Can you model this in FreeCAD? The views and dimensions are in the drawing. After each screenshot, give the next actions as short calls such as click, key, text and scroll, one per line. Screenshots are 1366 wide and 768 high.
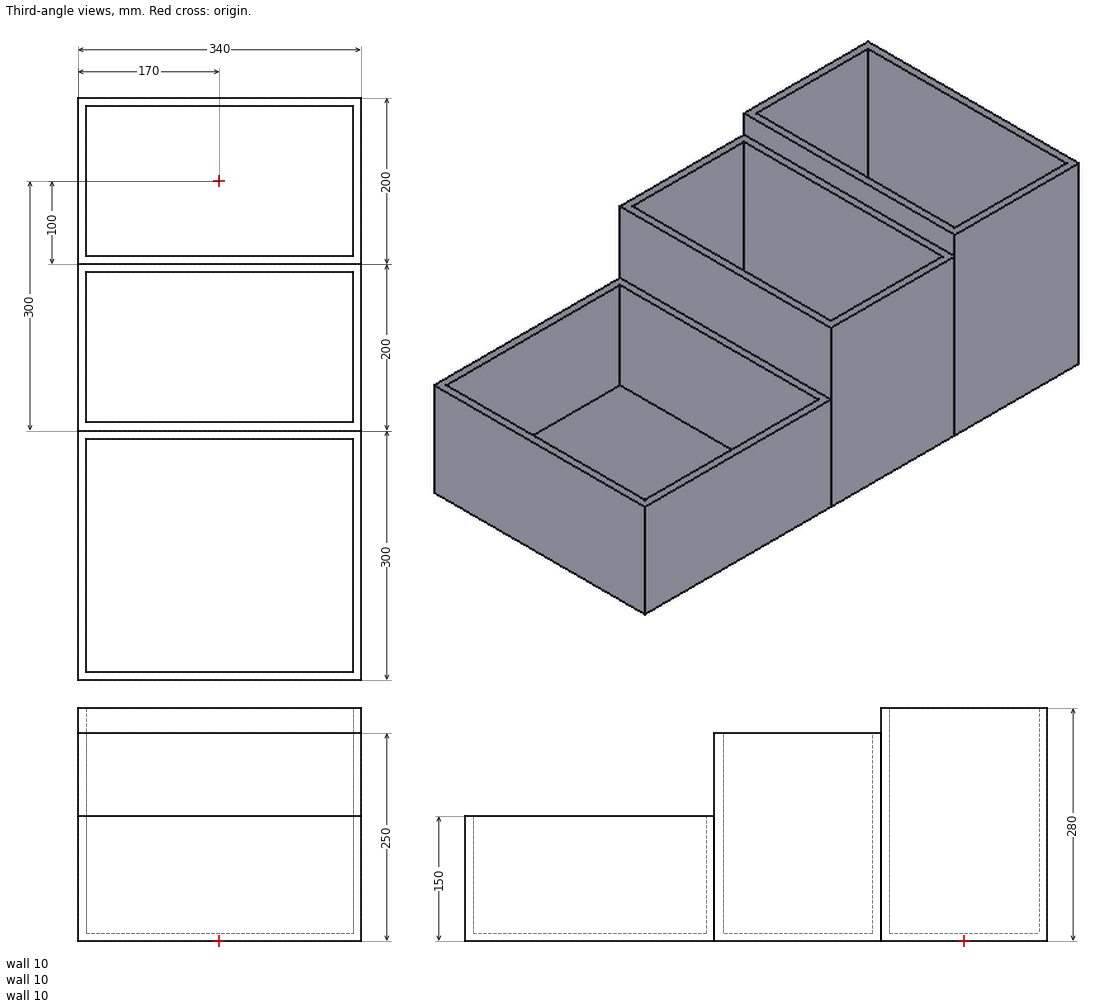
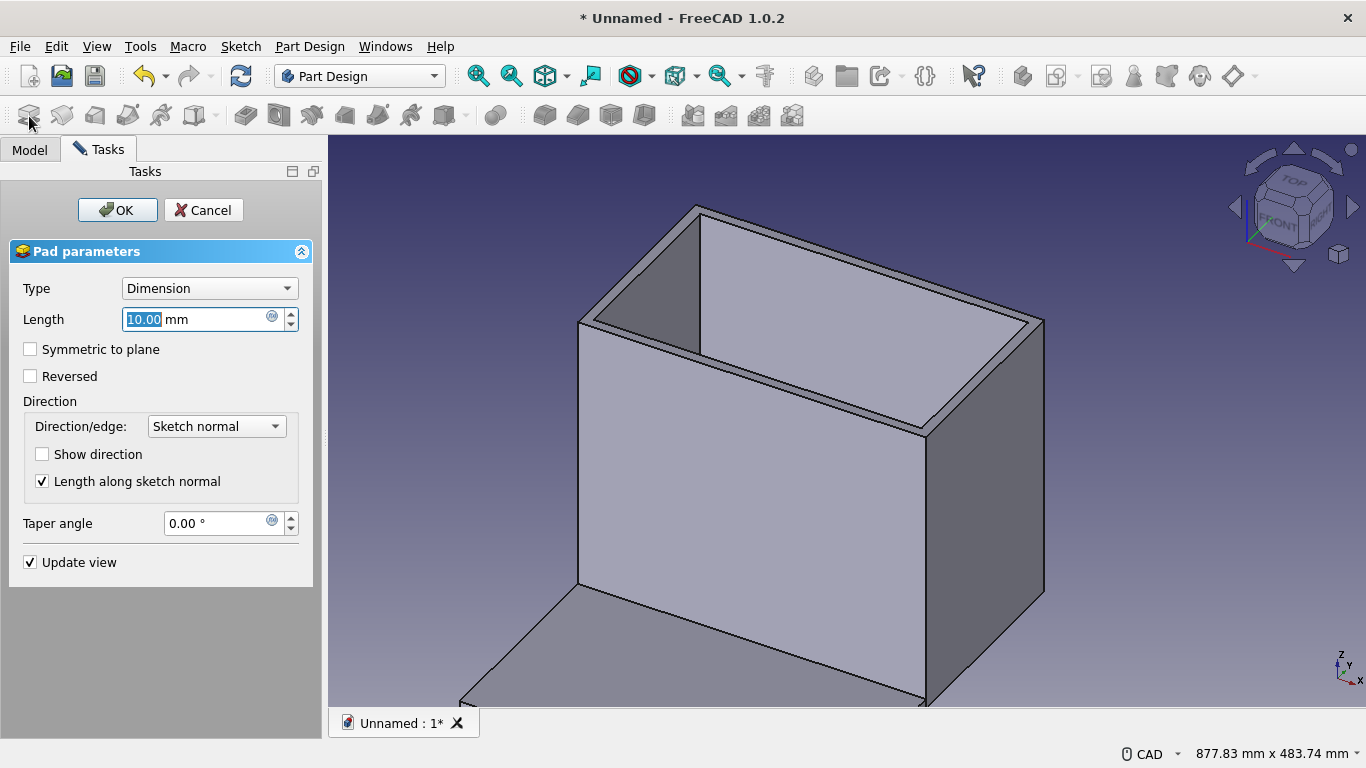
text(250)
key(Tab)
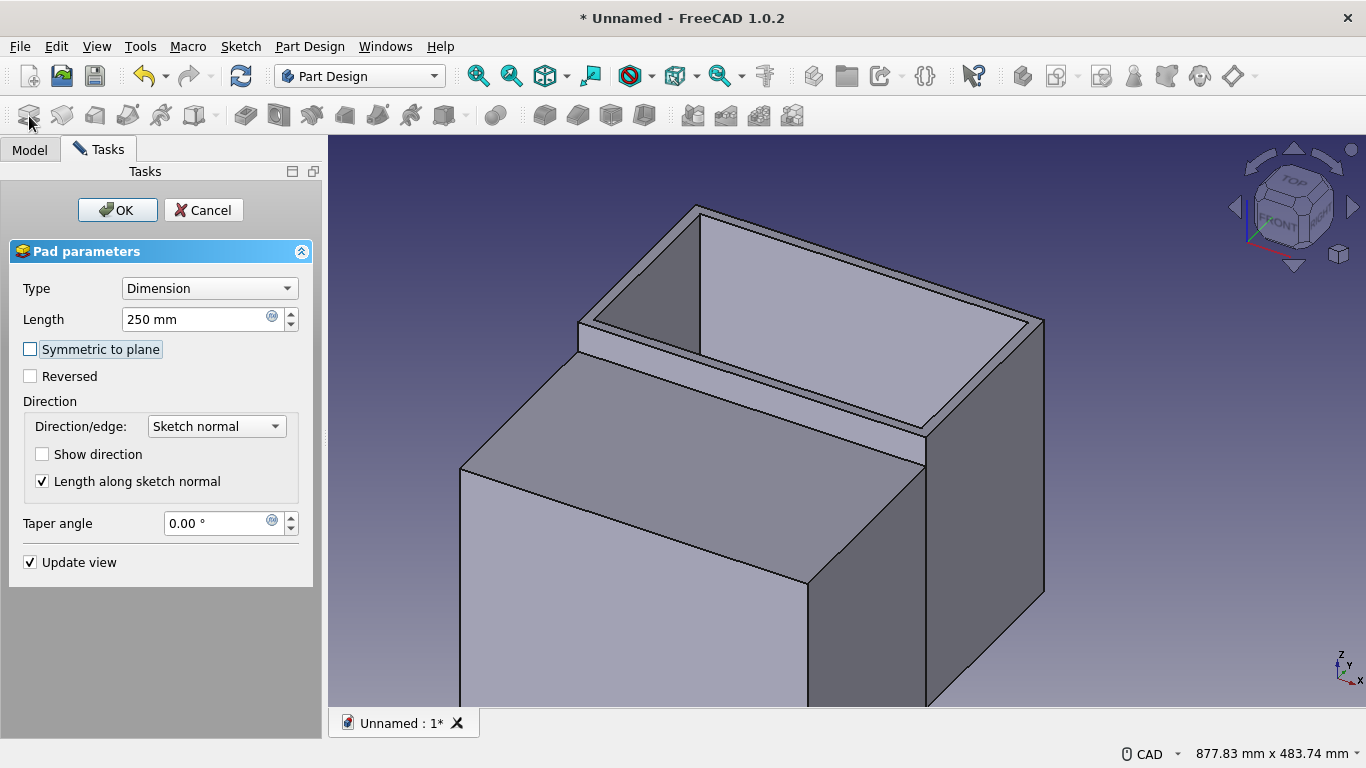
click(118, 210)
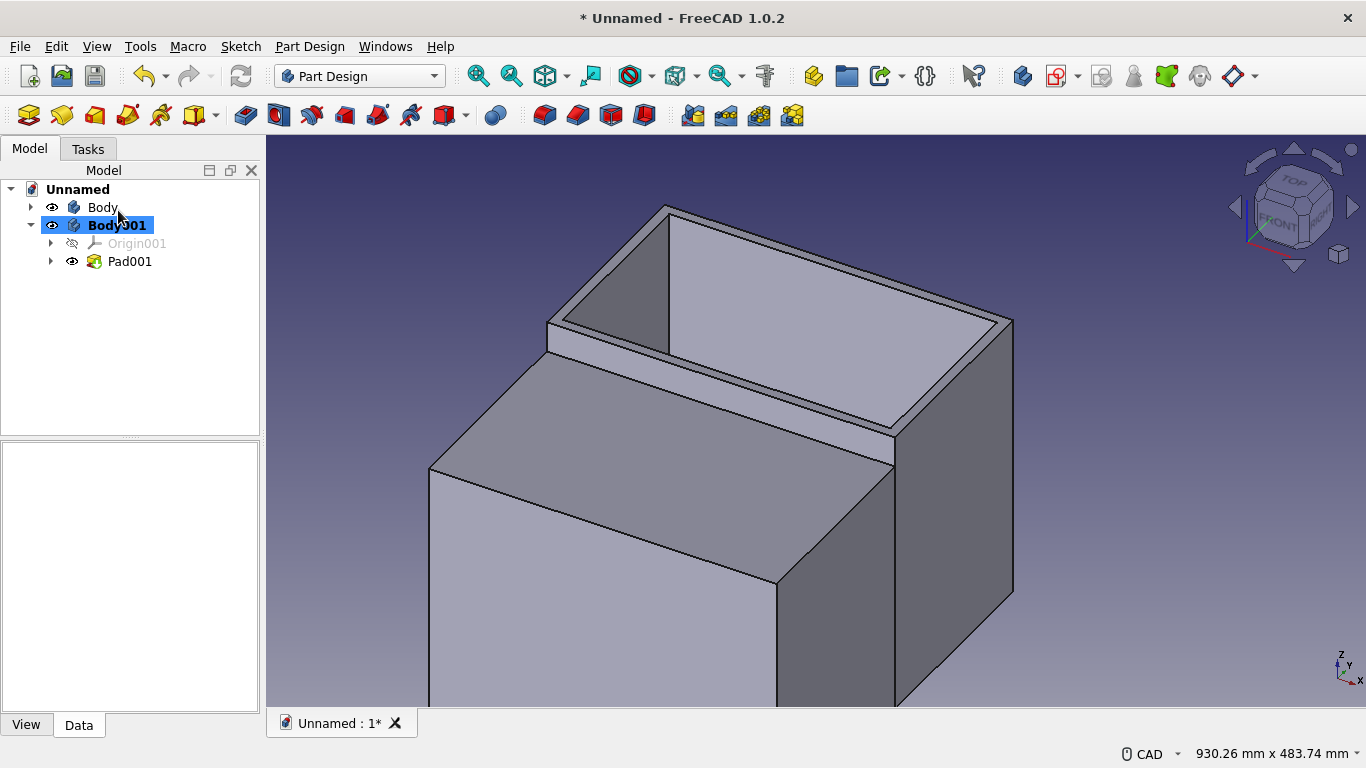
key(v)
key(f)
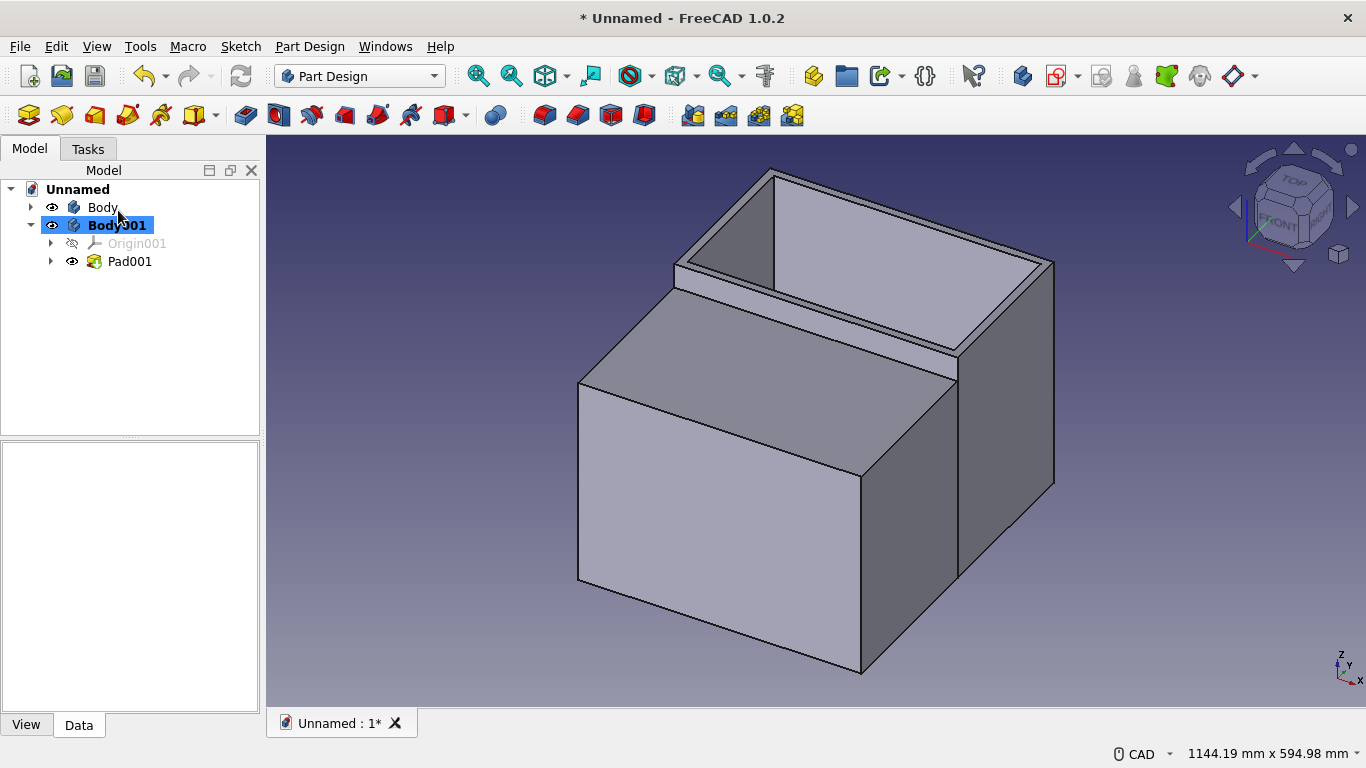
click(808, 395)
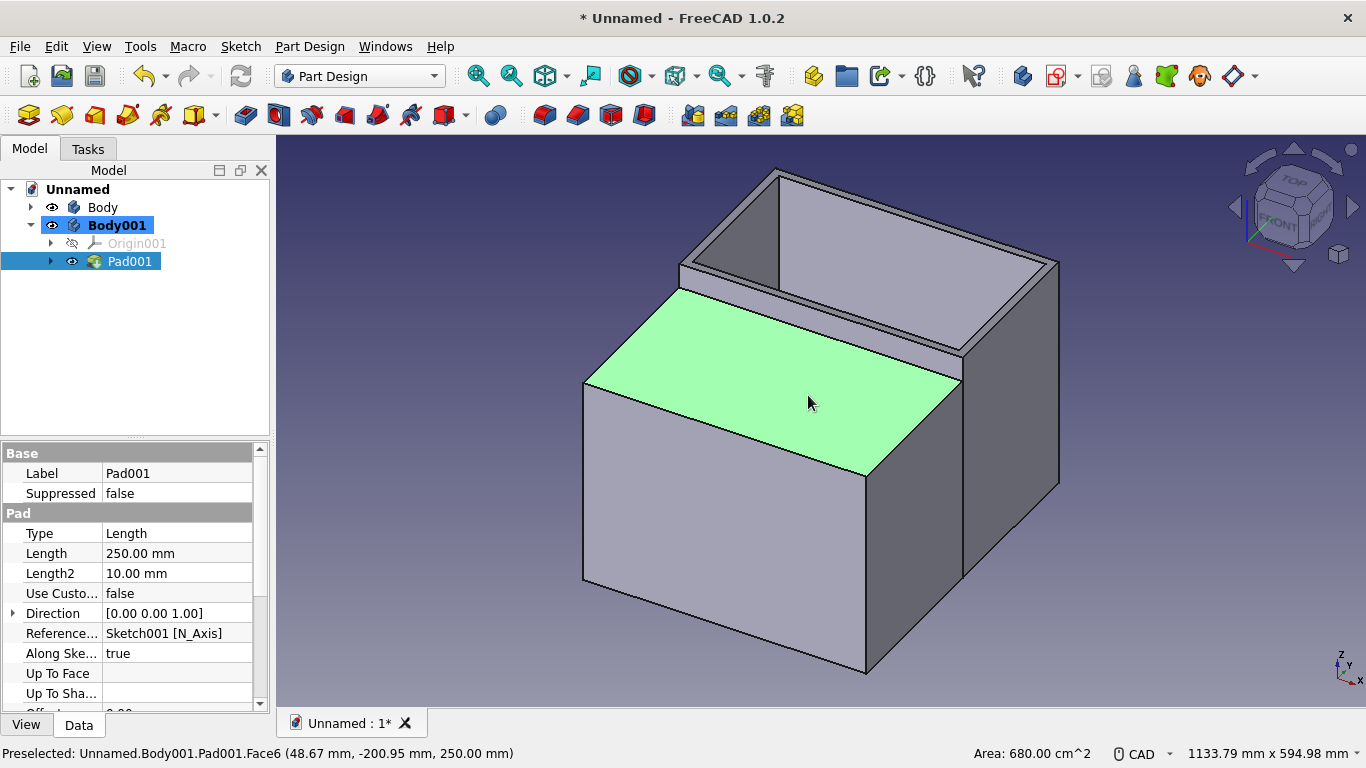
click(644, 116)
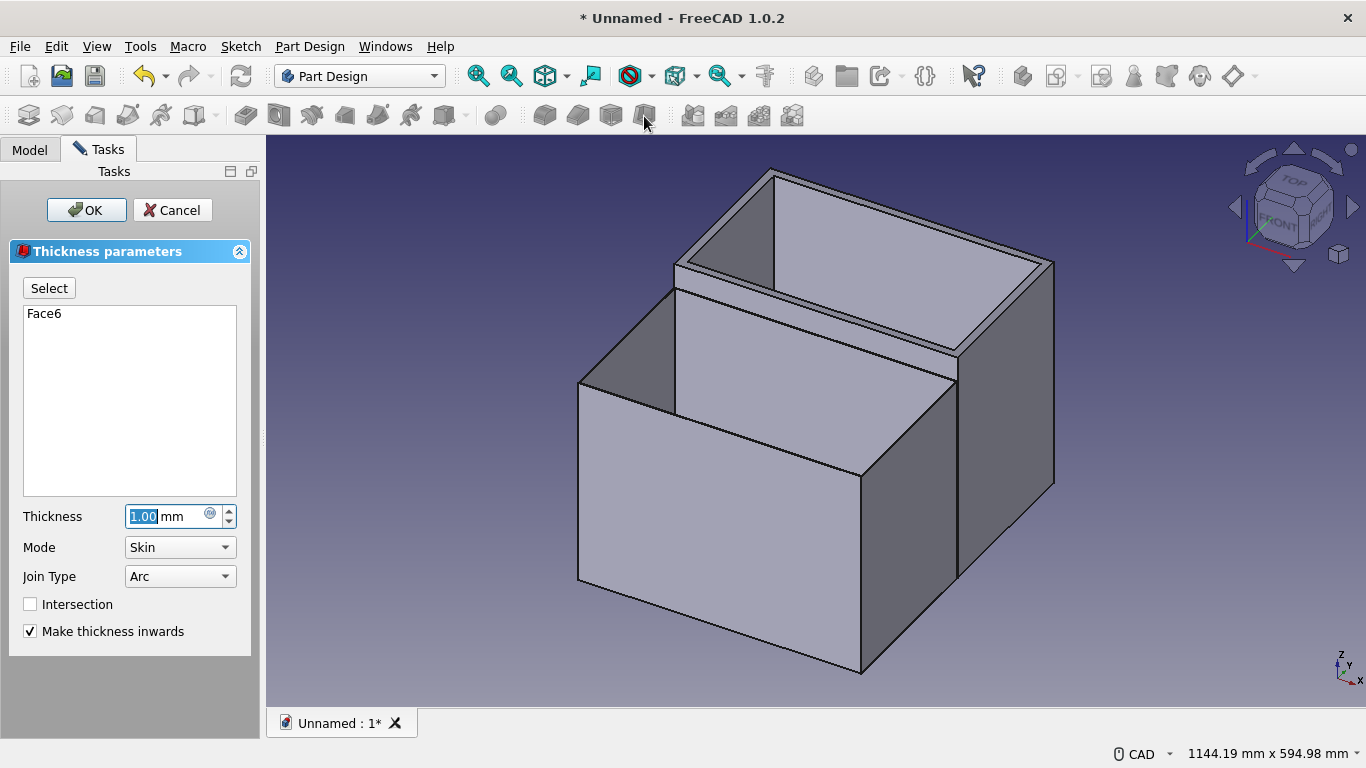
text(10)
key(Tab)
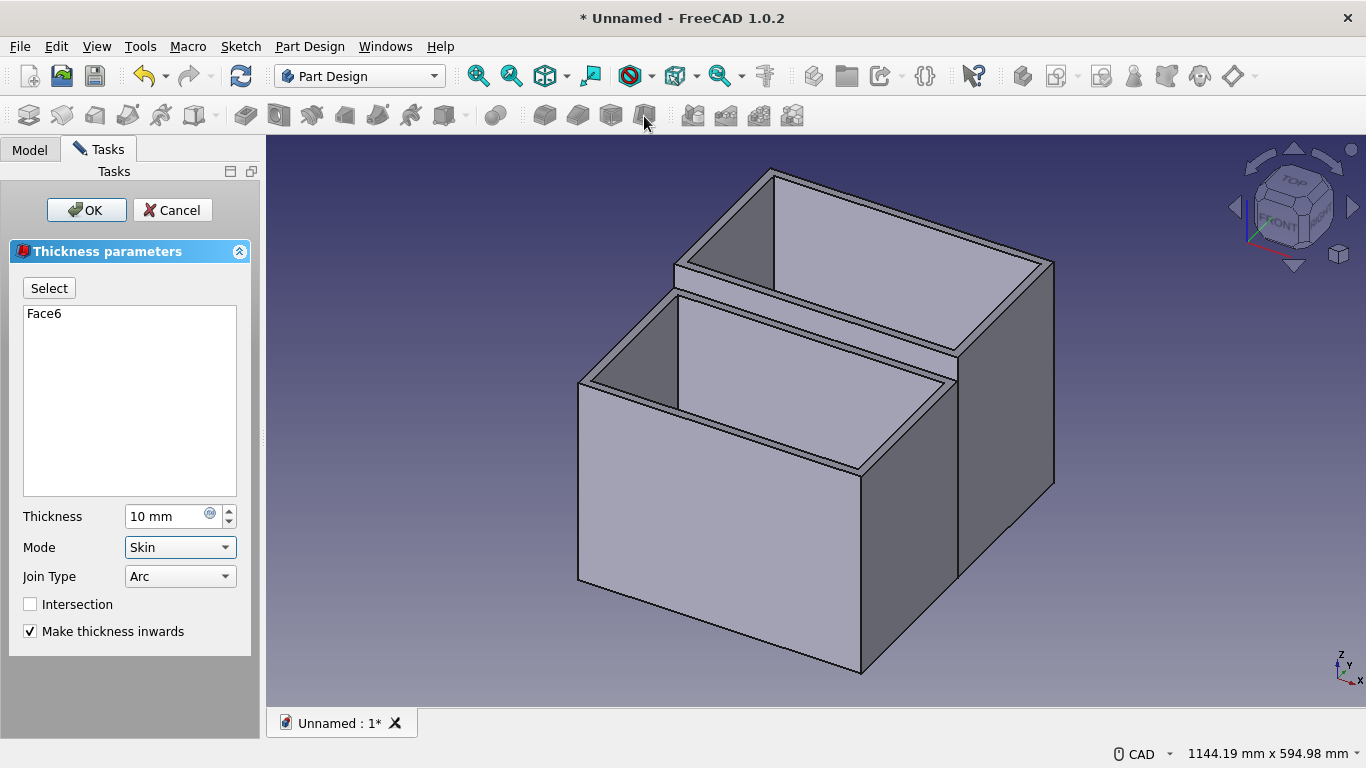
click(181, 576)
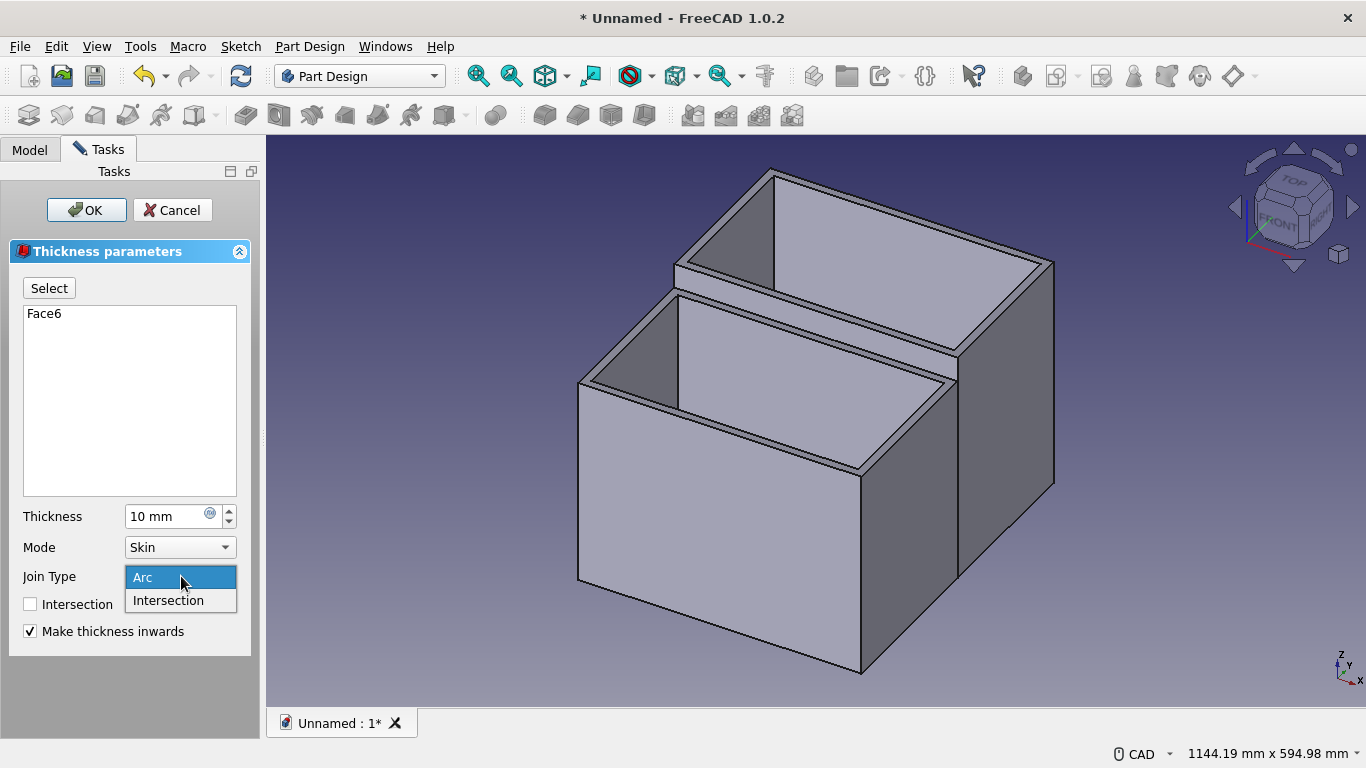
click(179, 600)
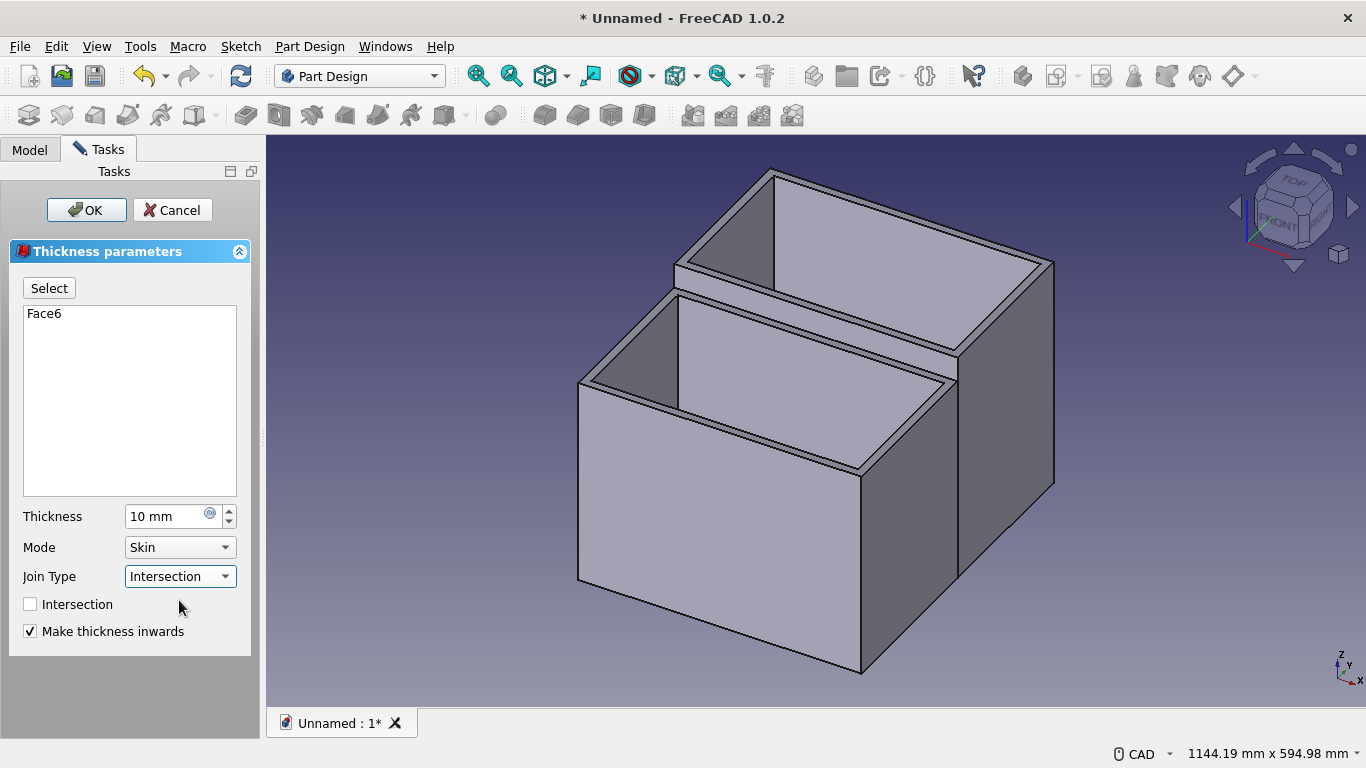
click(87, 210)